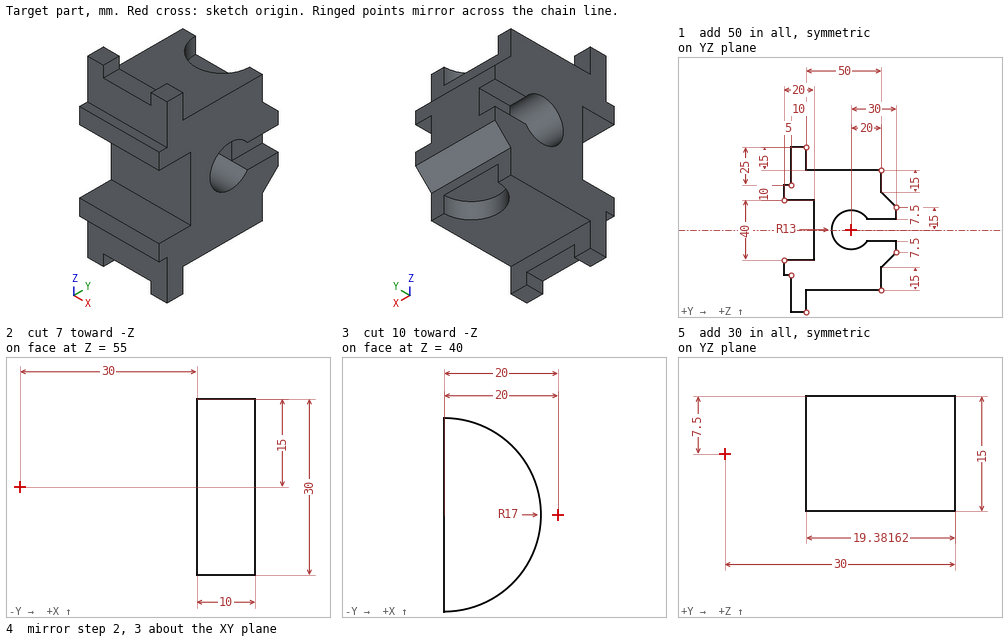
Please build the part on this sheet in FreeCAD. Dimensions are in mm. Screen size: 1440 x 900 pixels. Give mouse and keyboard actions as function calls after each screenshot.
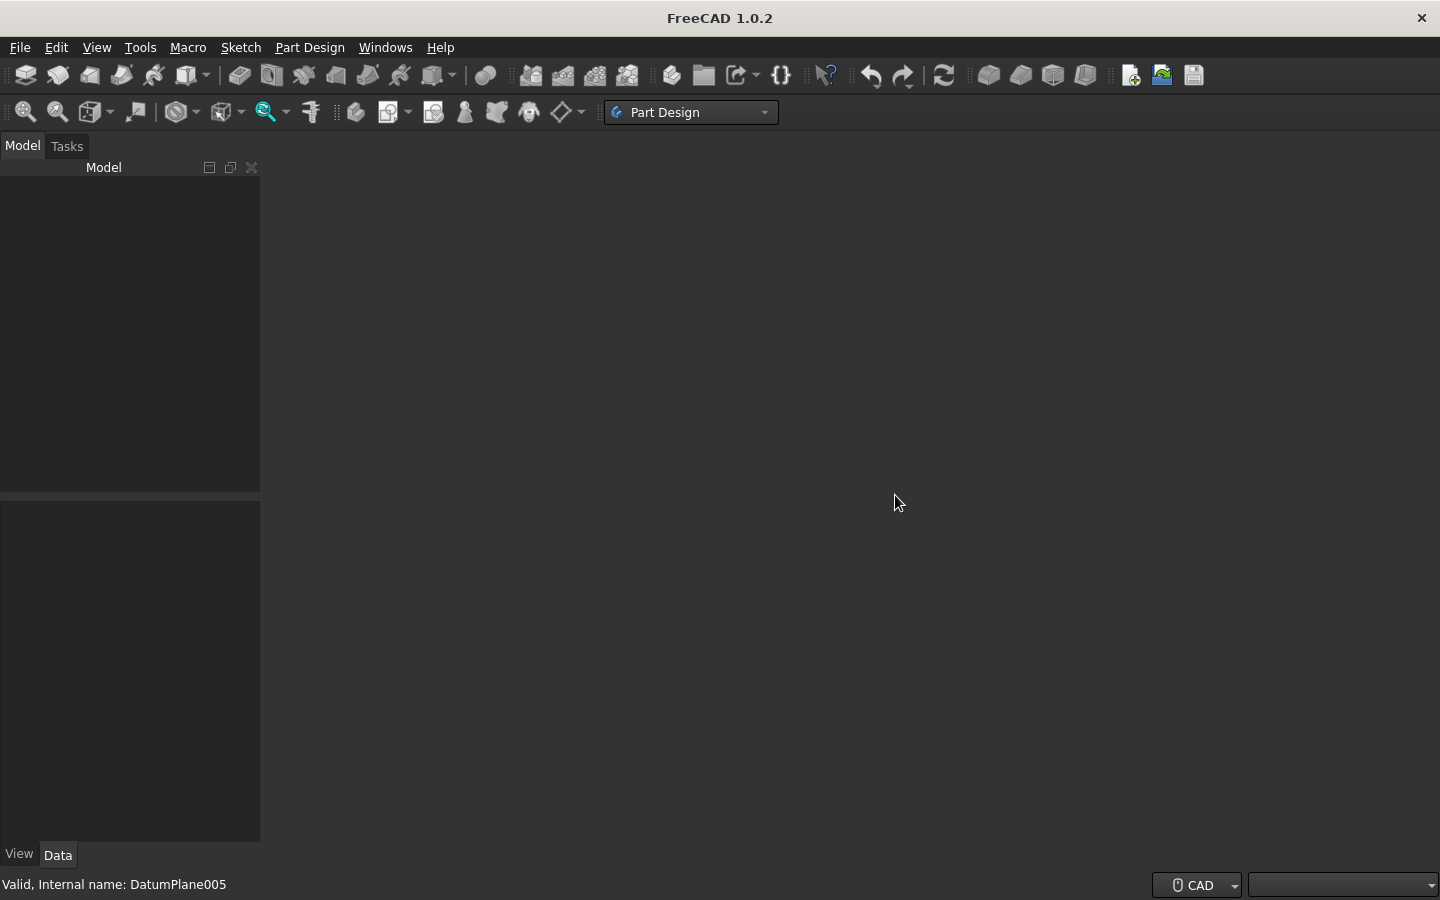
click(1130, 76)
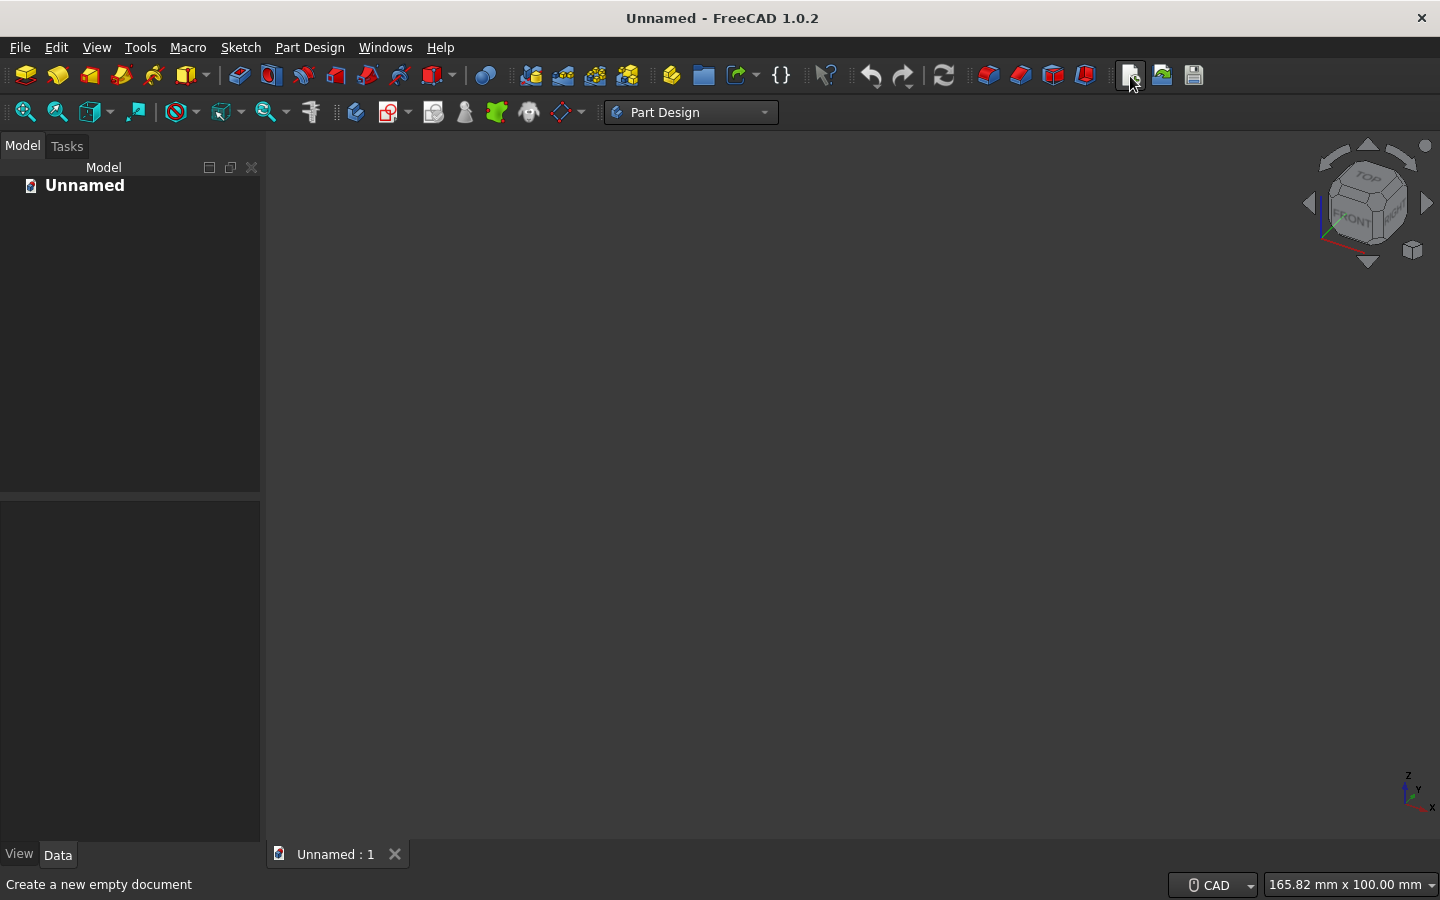
click(388, 112)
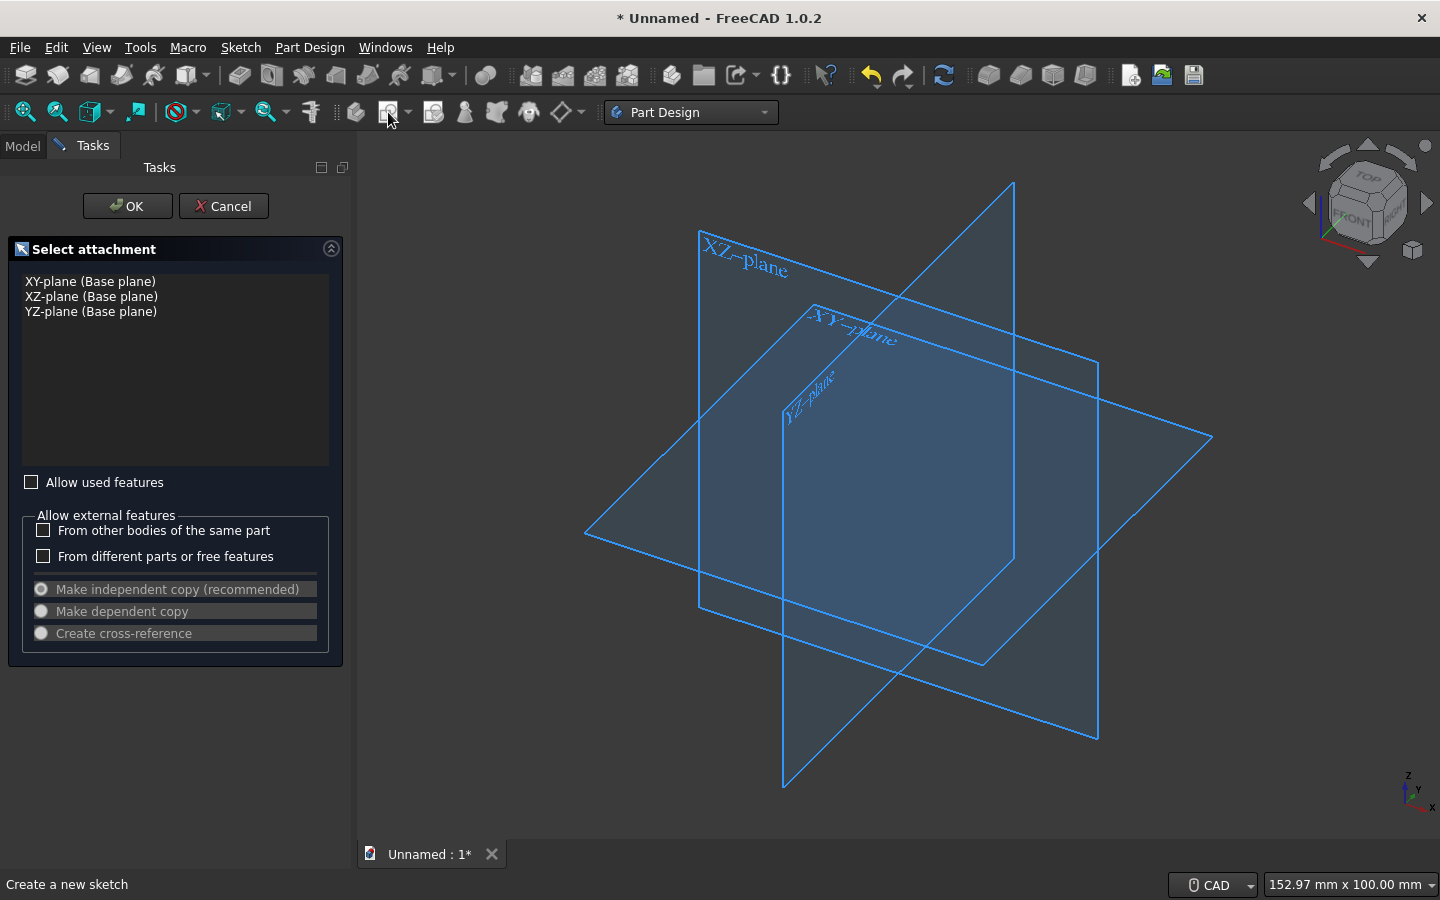
click(82, 312)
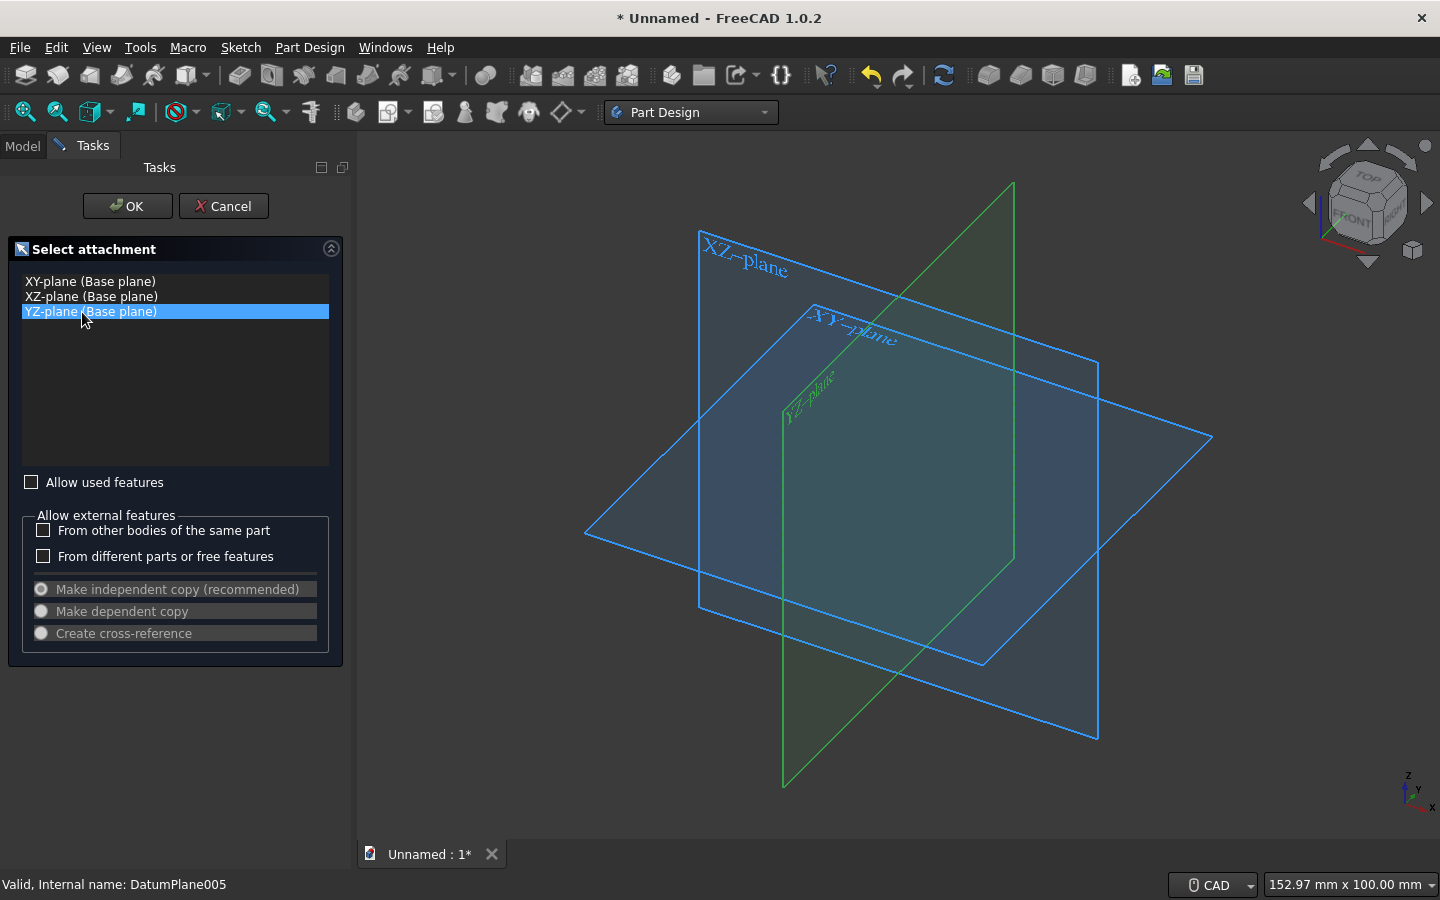
click(128, 206)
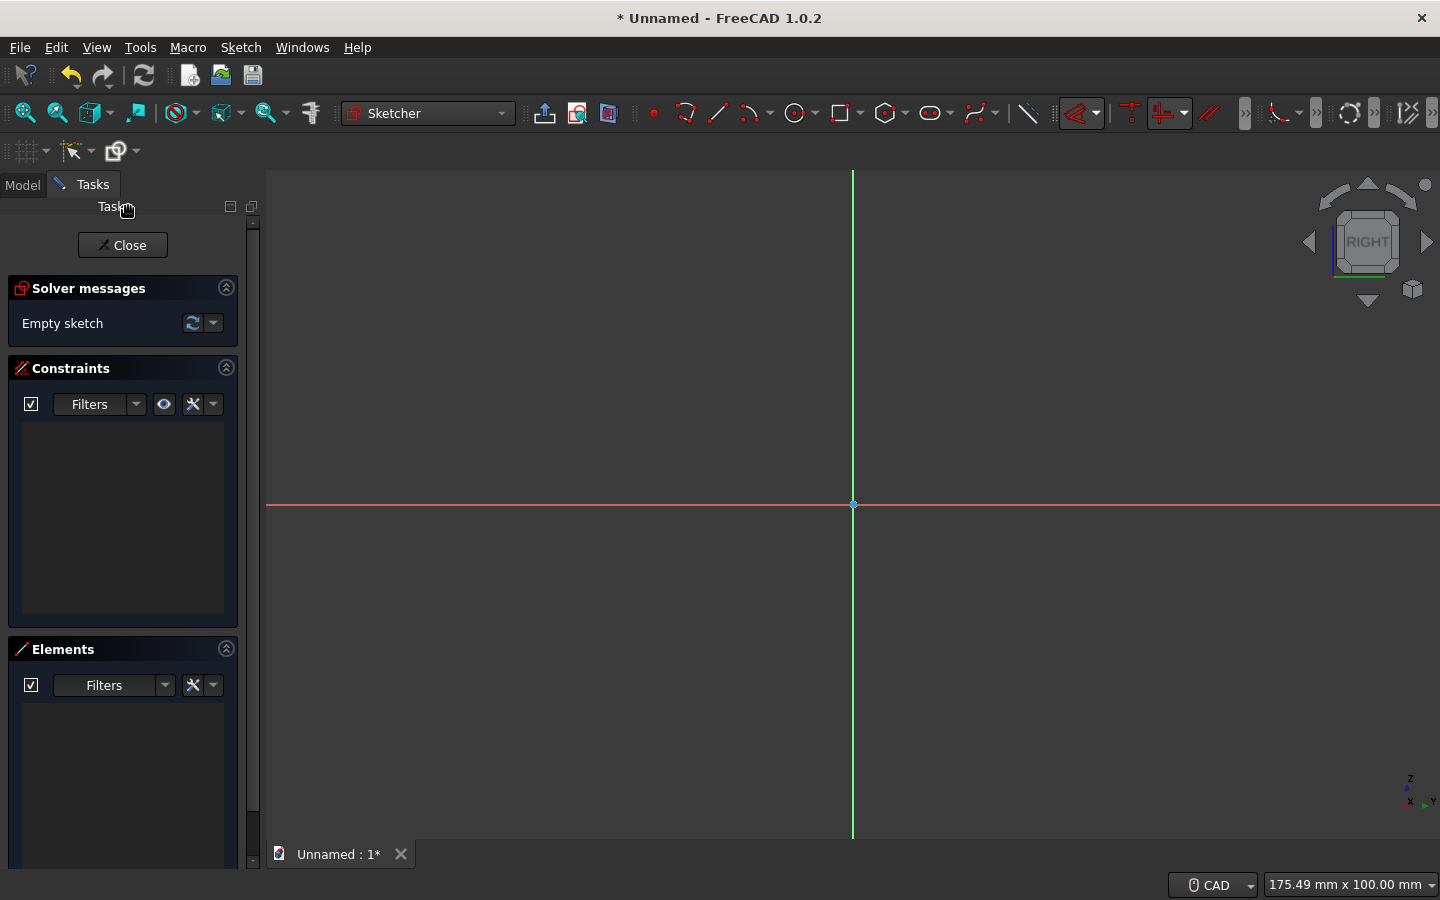
scroll(762, 504, down, 3)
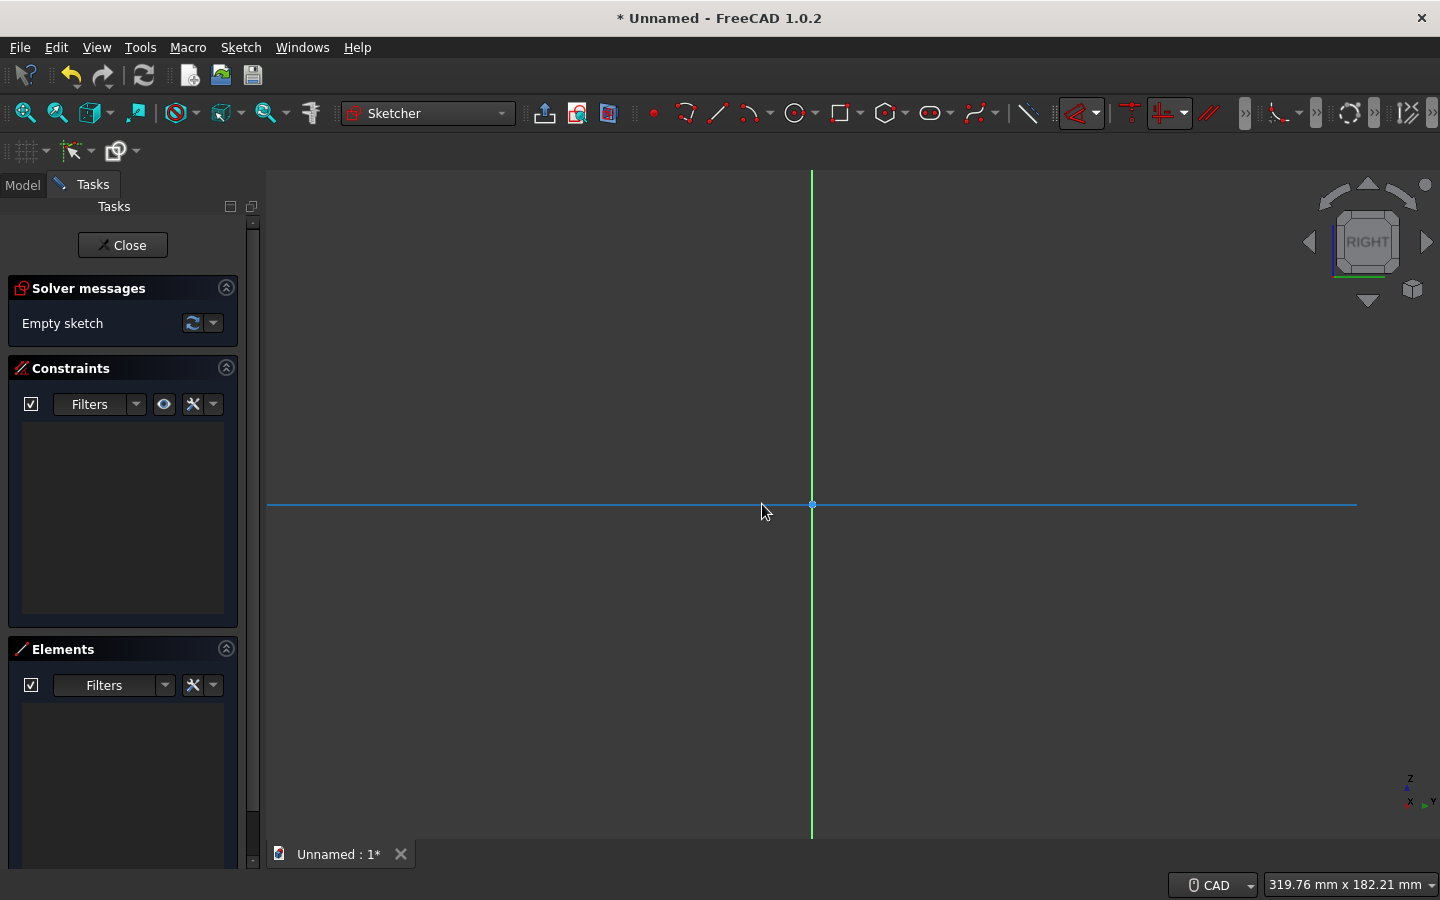
click(686, 114)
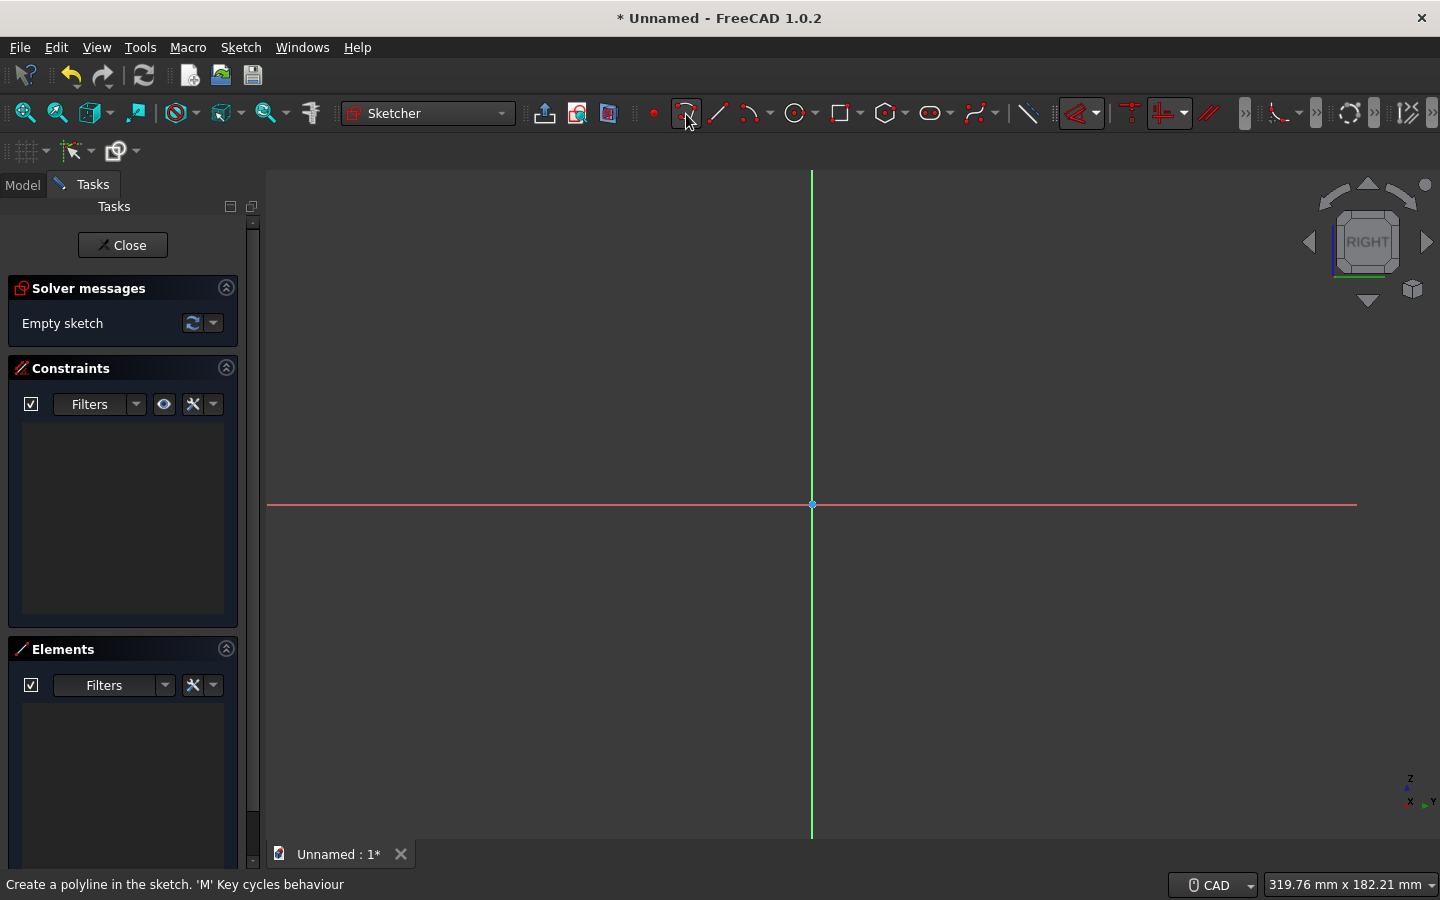
click(851, 477)
click(922, 477)
click(922, 449)
click(886, 413)
click(886, 358)
click(702, 358)
click(702, 303)
click(665, 303)
click(665, 394)
click(647, 394)
click(647, 431)
click(720, 431)
click(720, 578)
click(647, 578)
click(647, 615)
click(665, 615)
click(665, 706)
click(702, 706)
click(702, 651)
click(886, 651)
click(886, 596)
click(922, 560)
click(922, 532)
click(851, 532)
right_click(851, 532)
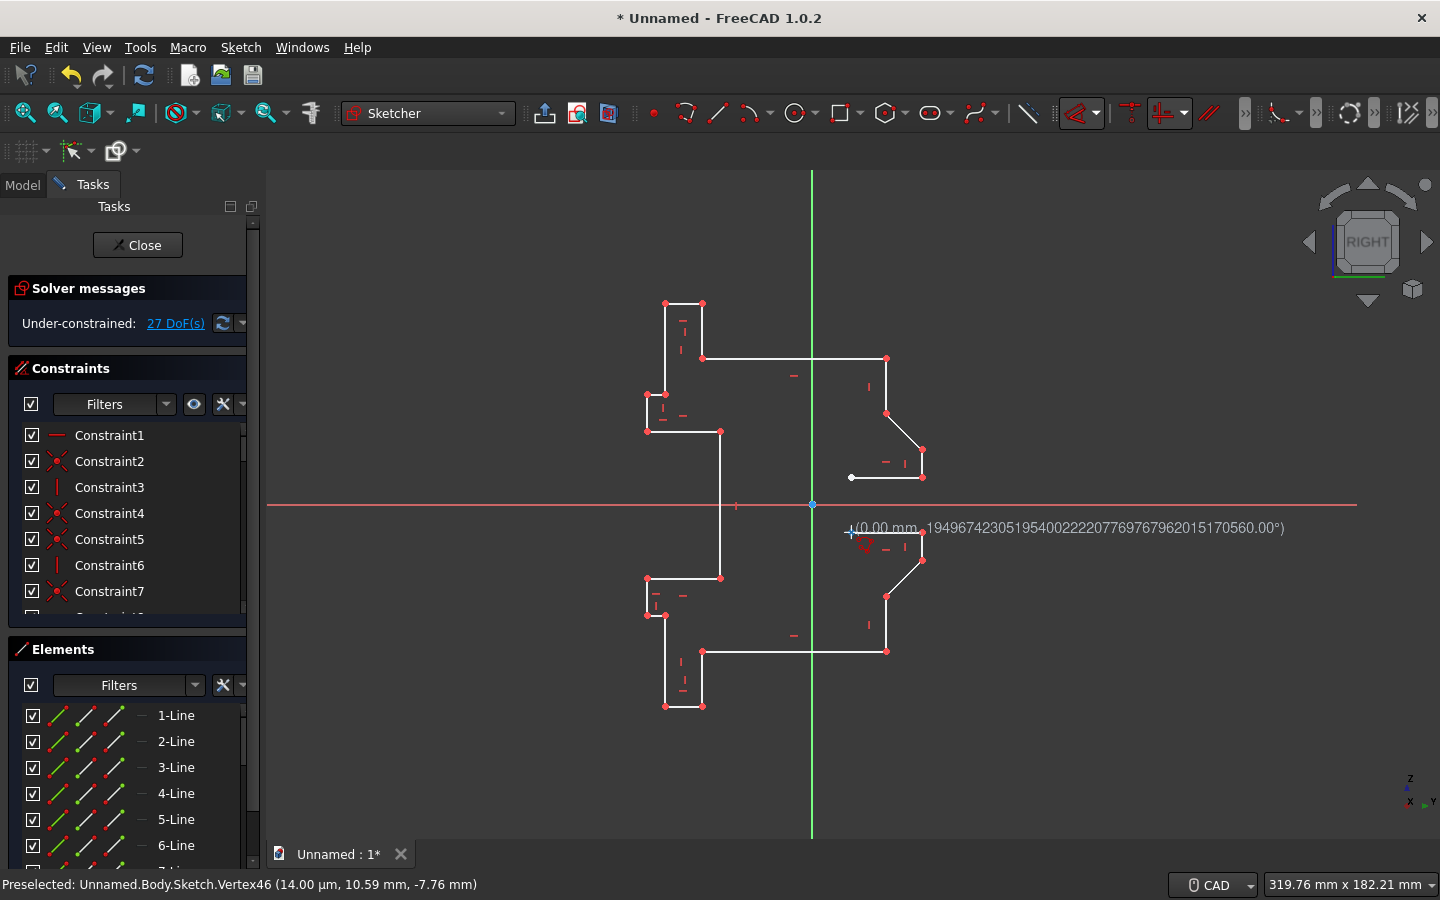
key(g)
key(3)
key(a)